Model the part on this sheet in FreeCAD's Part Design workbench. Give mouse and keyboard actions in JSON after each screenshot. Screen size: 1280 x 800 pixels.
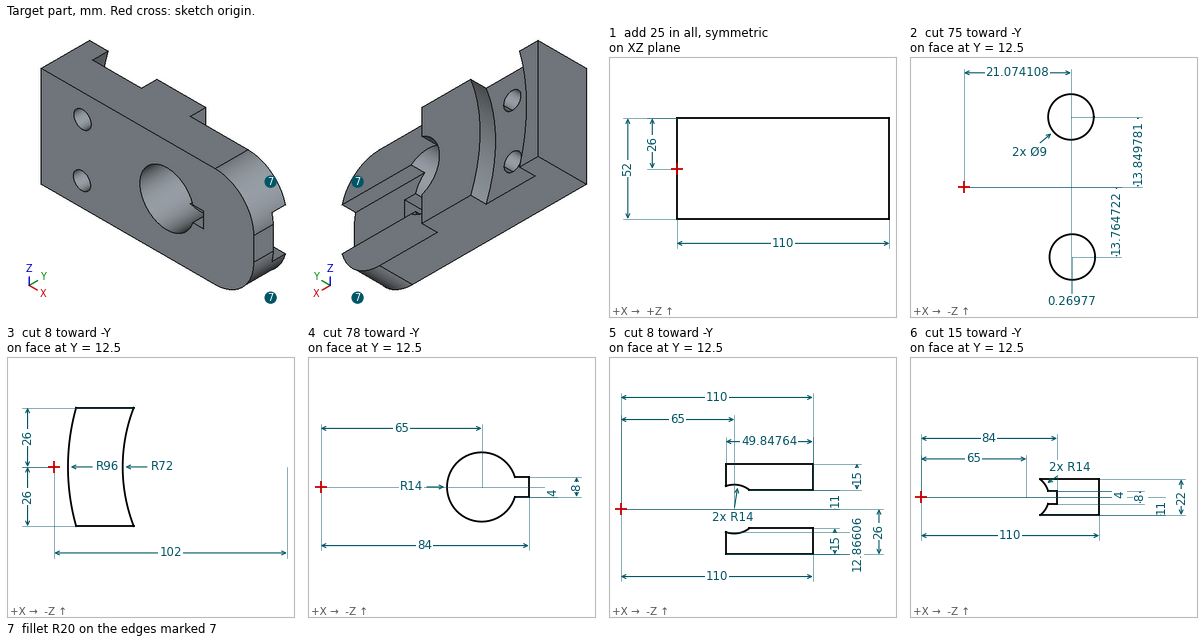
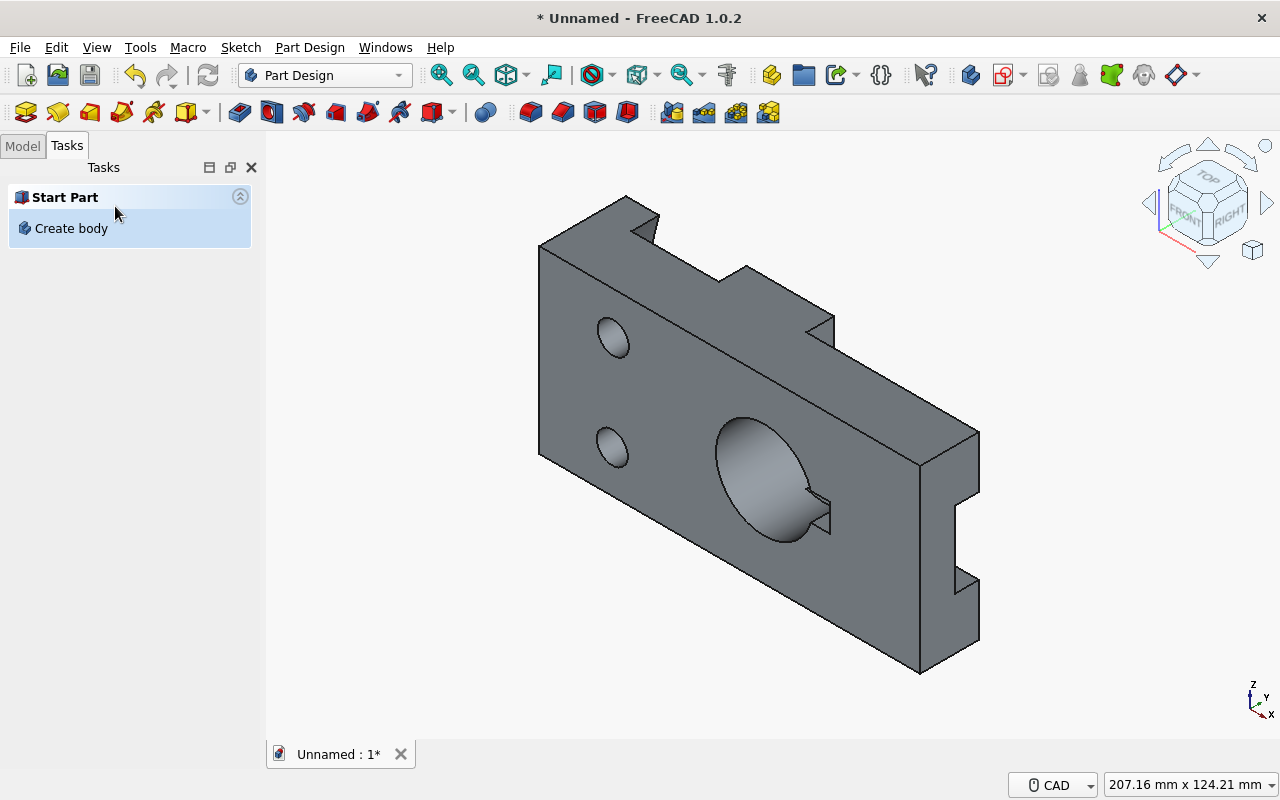
{"action": "left_click", "coordinate": [950, 448]}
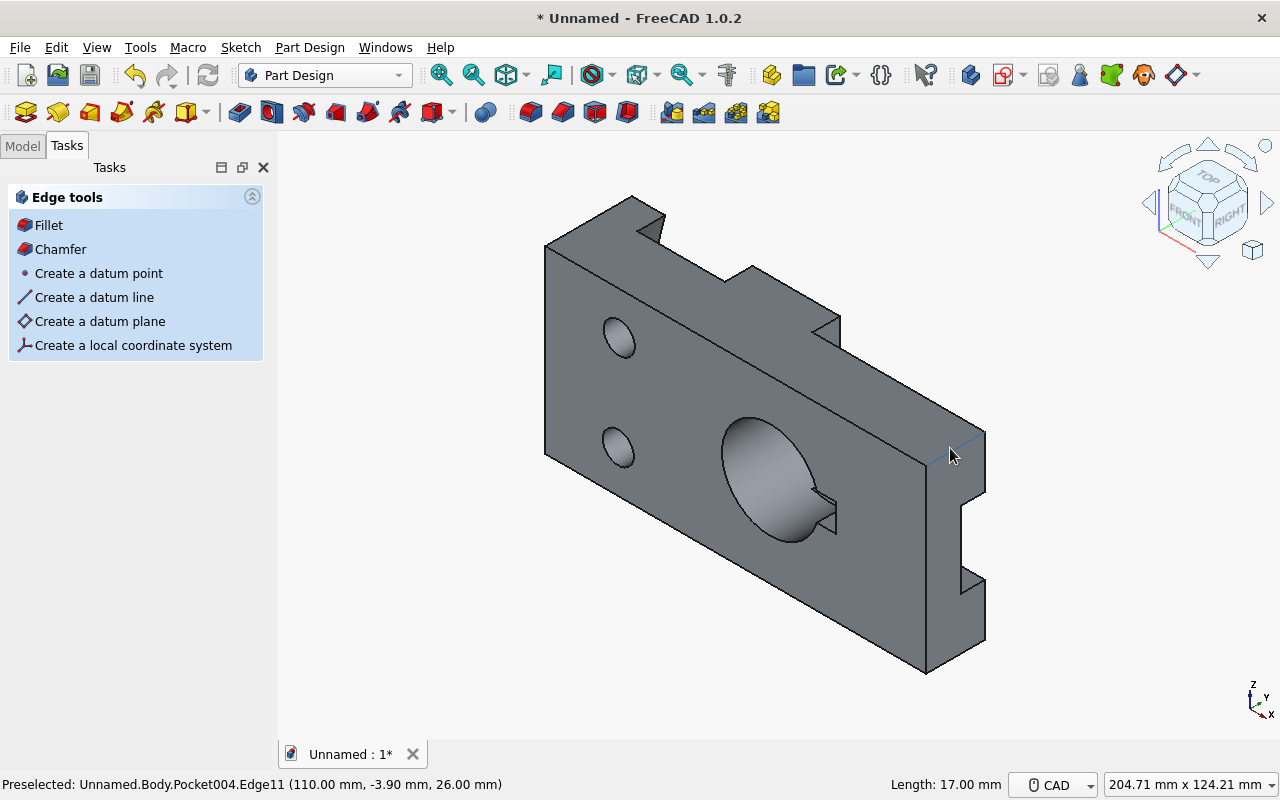
{"action": "key", "text": "2"}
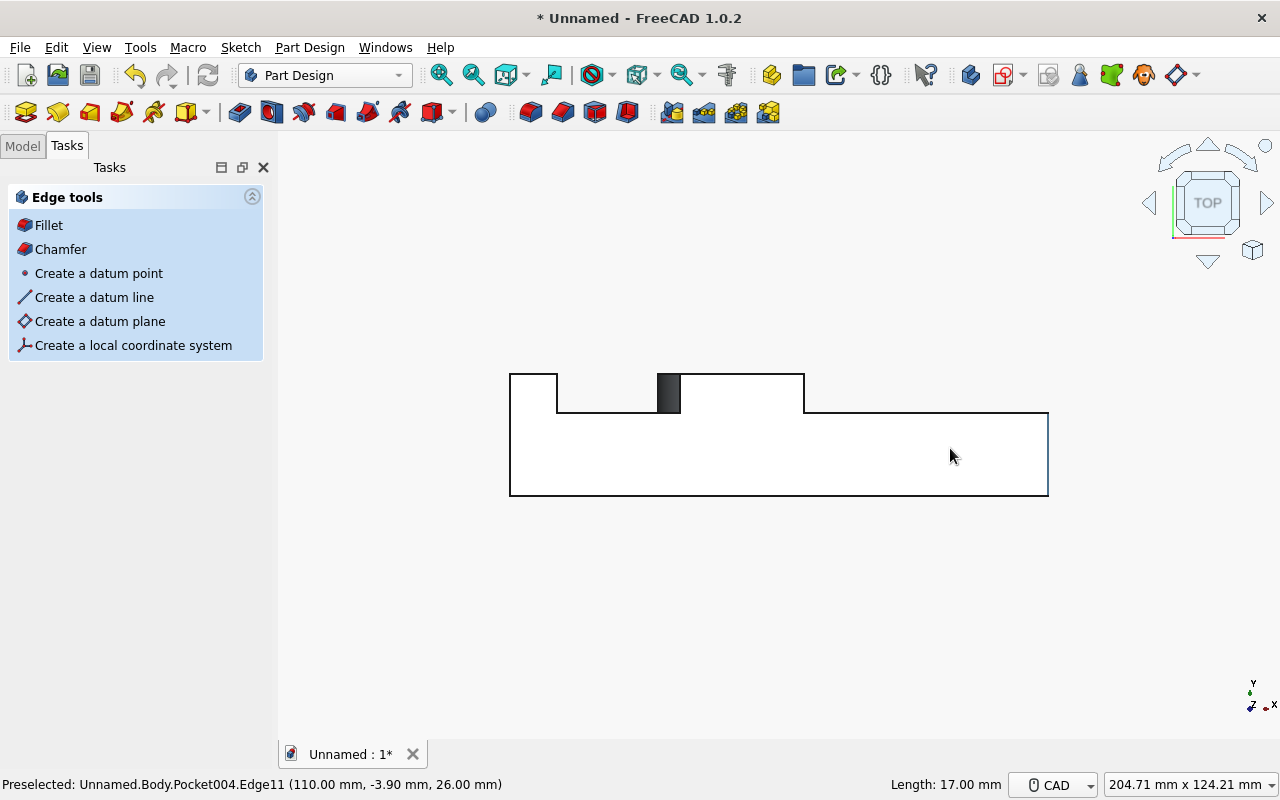
{"action": "key", "text": "1"}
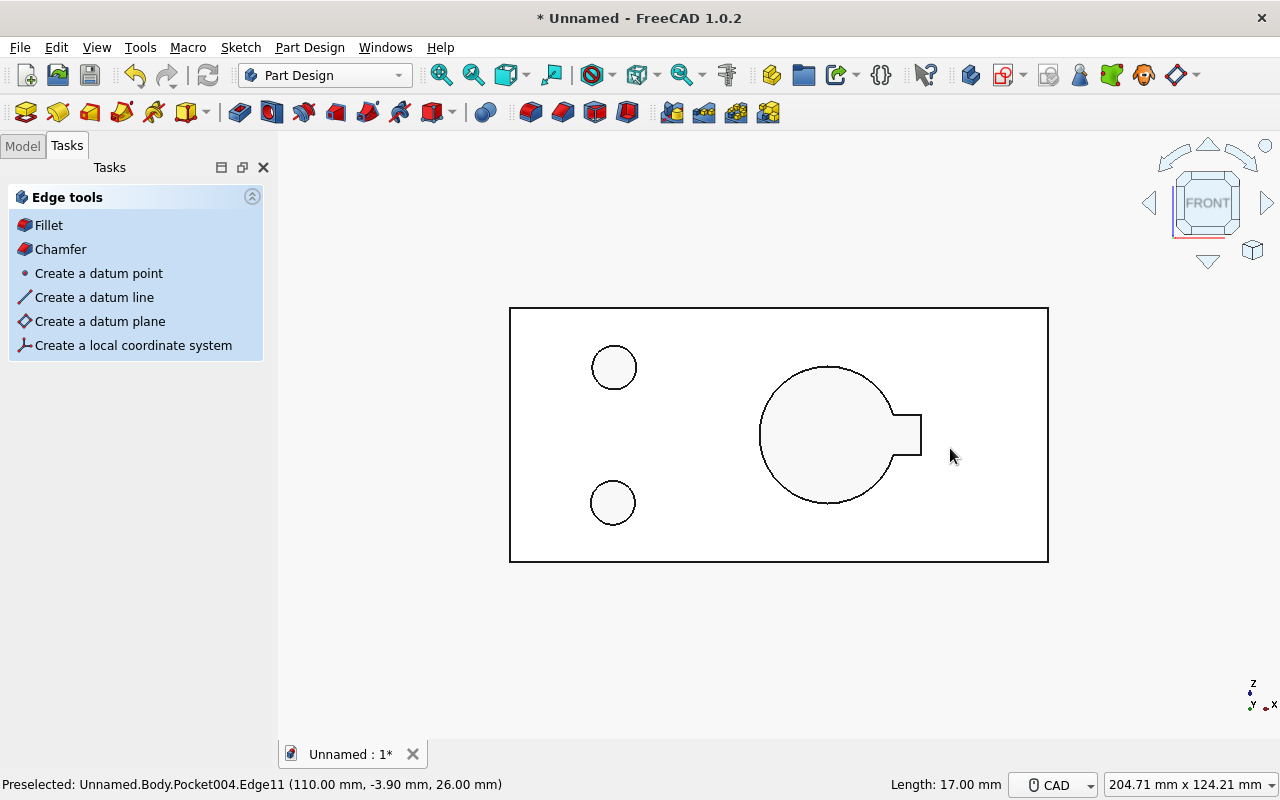
{"action": "key", "text": "3"}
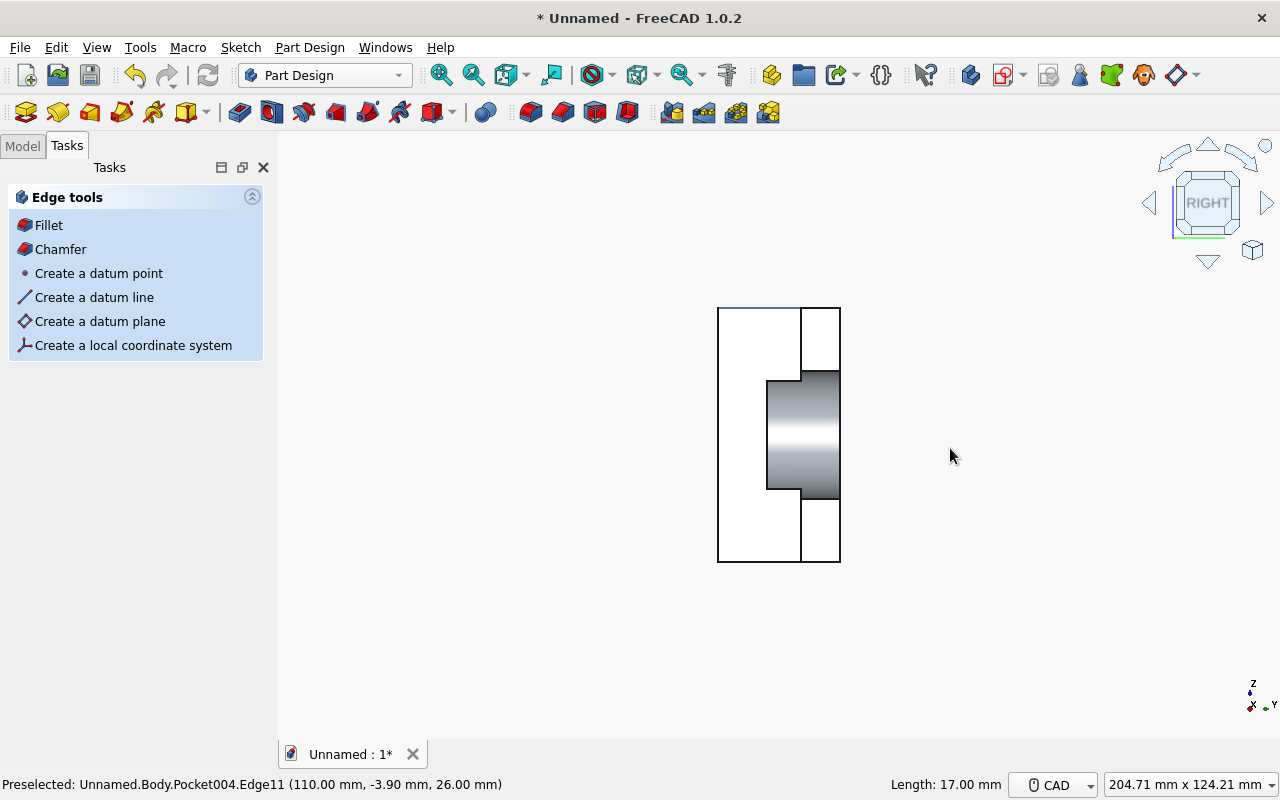
{"action": "left_click", "coordinate": [442, 76]}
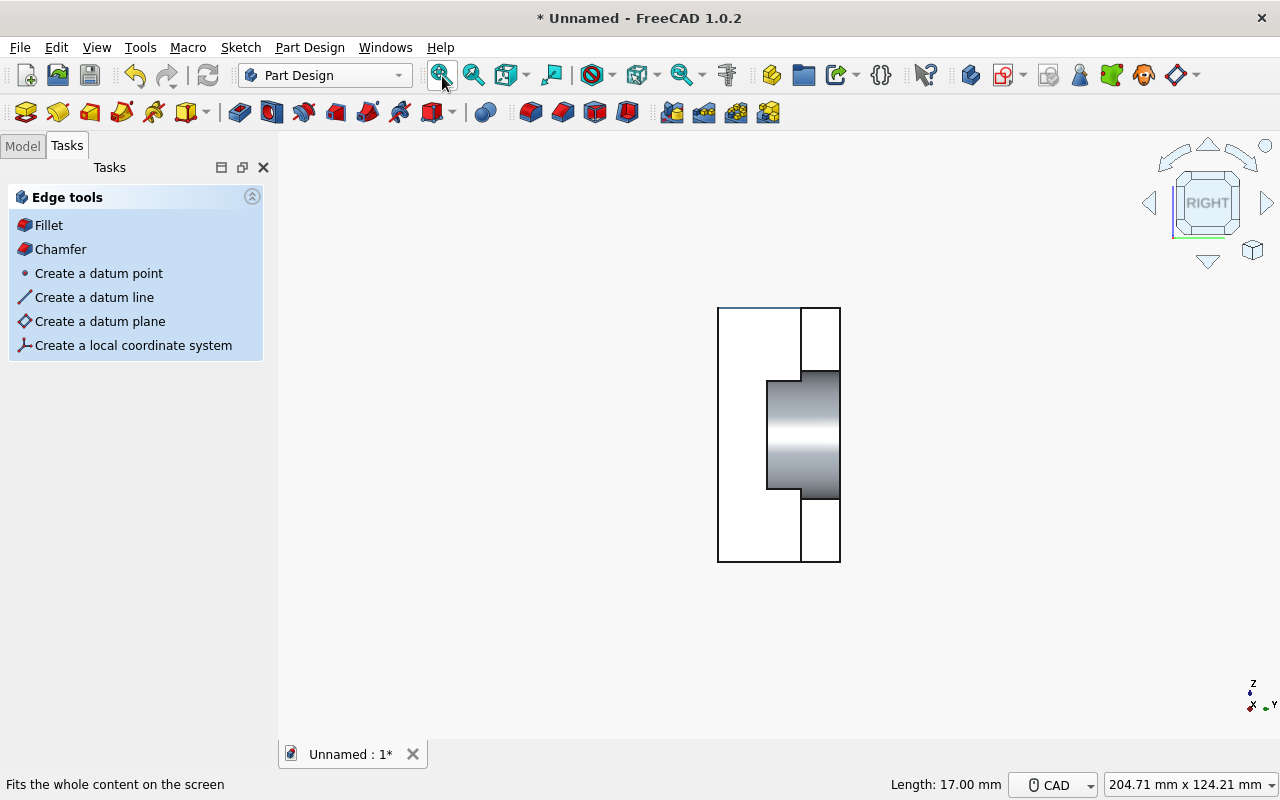
{"action": "left_click", "coordinate": [759, 561], "text": "ctrl"}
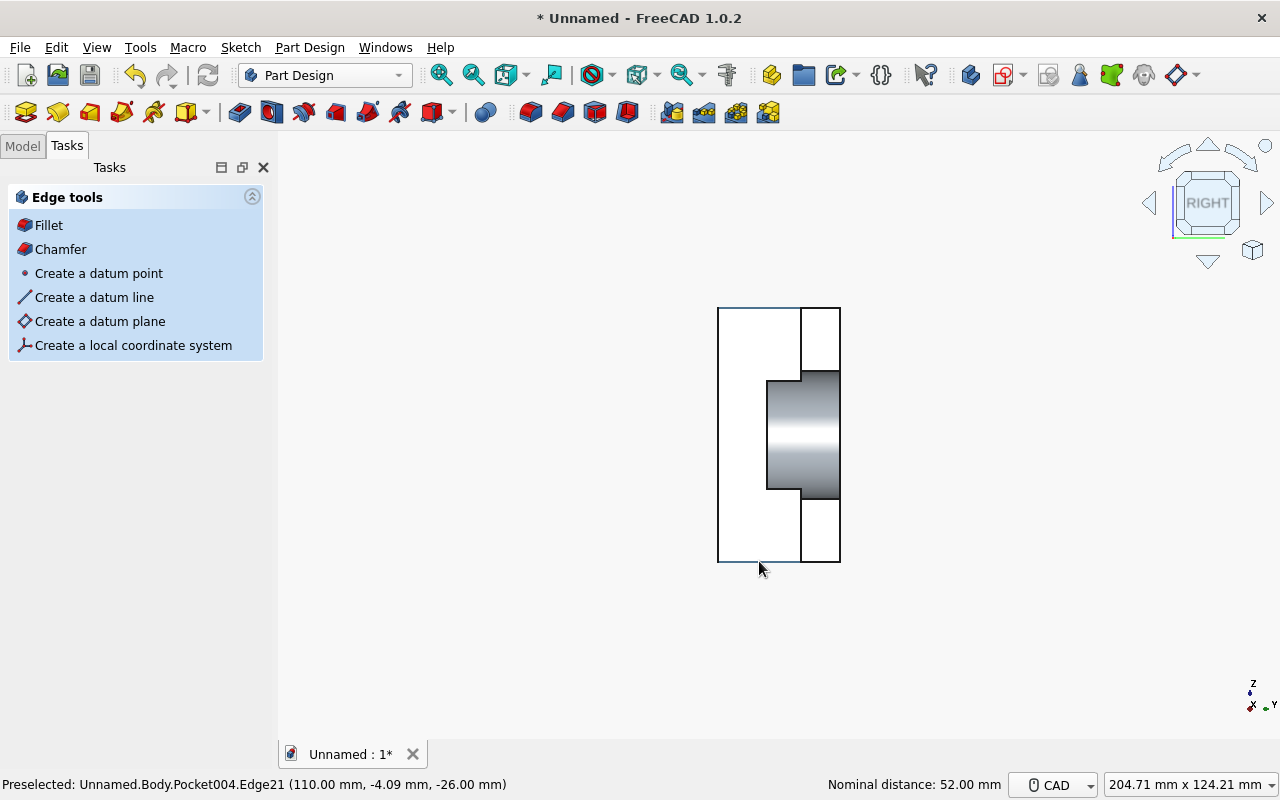
{"action": "left_click", "coordinate": [532, 112]}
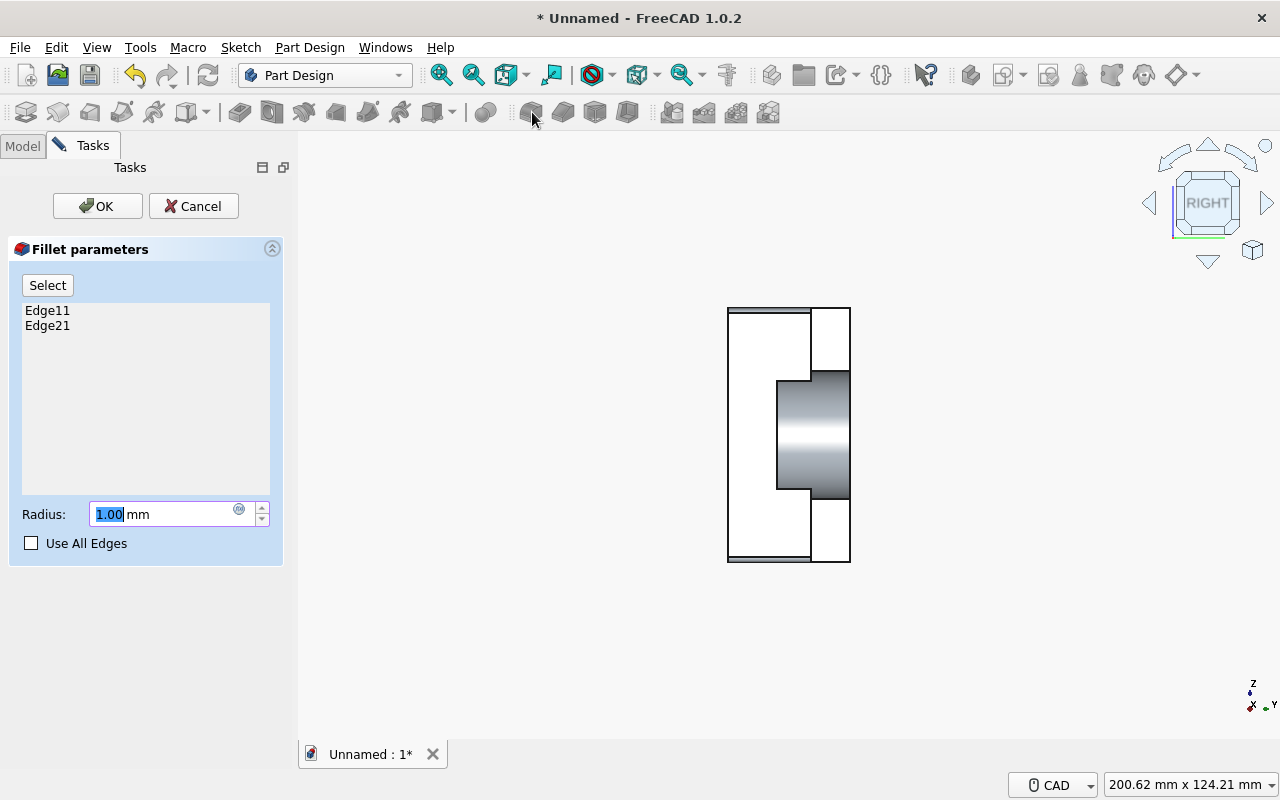
{"action": "type", "text": "20"}
{"action": "key", "text": "Tab"}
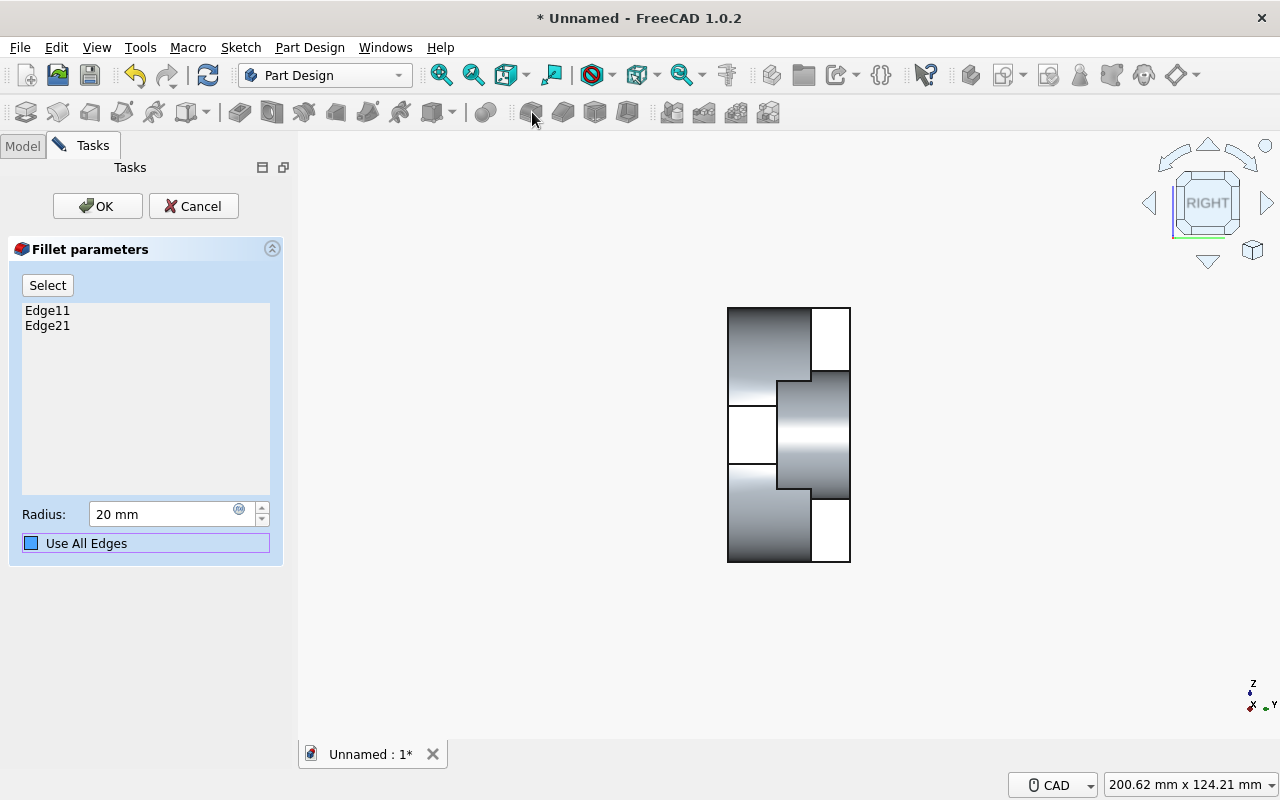
{"action": "left_click", "coordinate": [98, 206]}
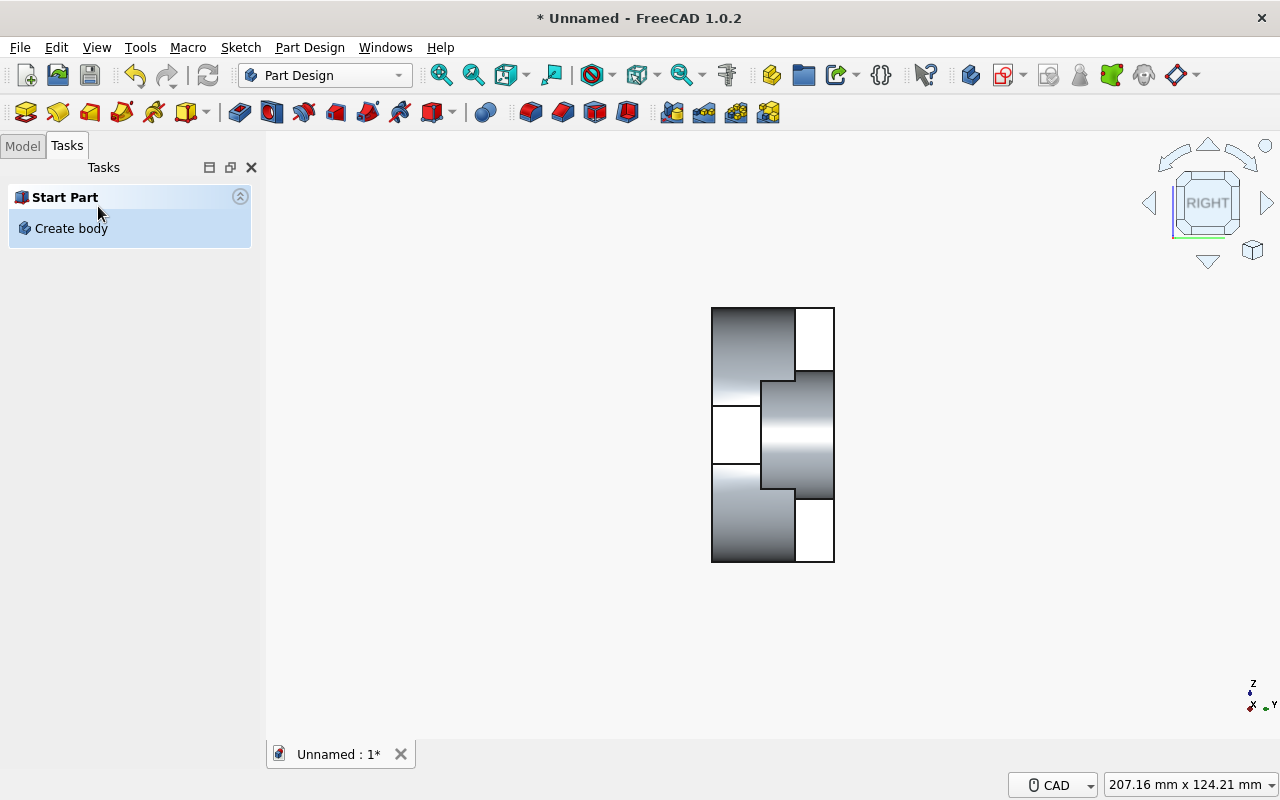
{"action": "key", "text": "0"}